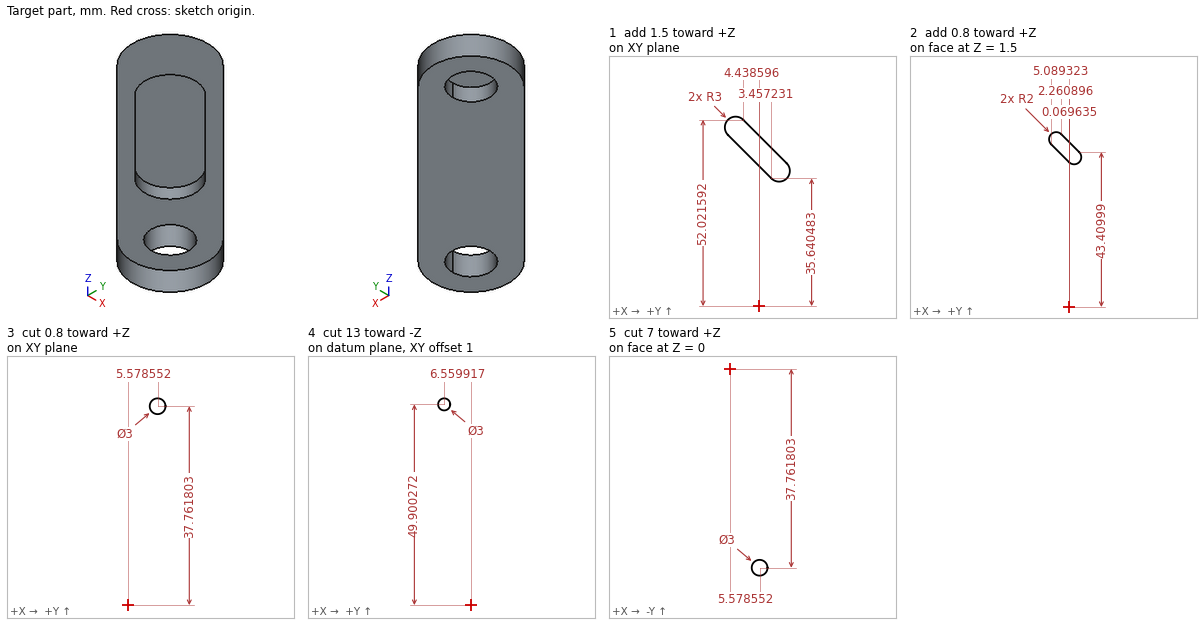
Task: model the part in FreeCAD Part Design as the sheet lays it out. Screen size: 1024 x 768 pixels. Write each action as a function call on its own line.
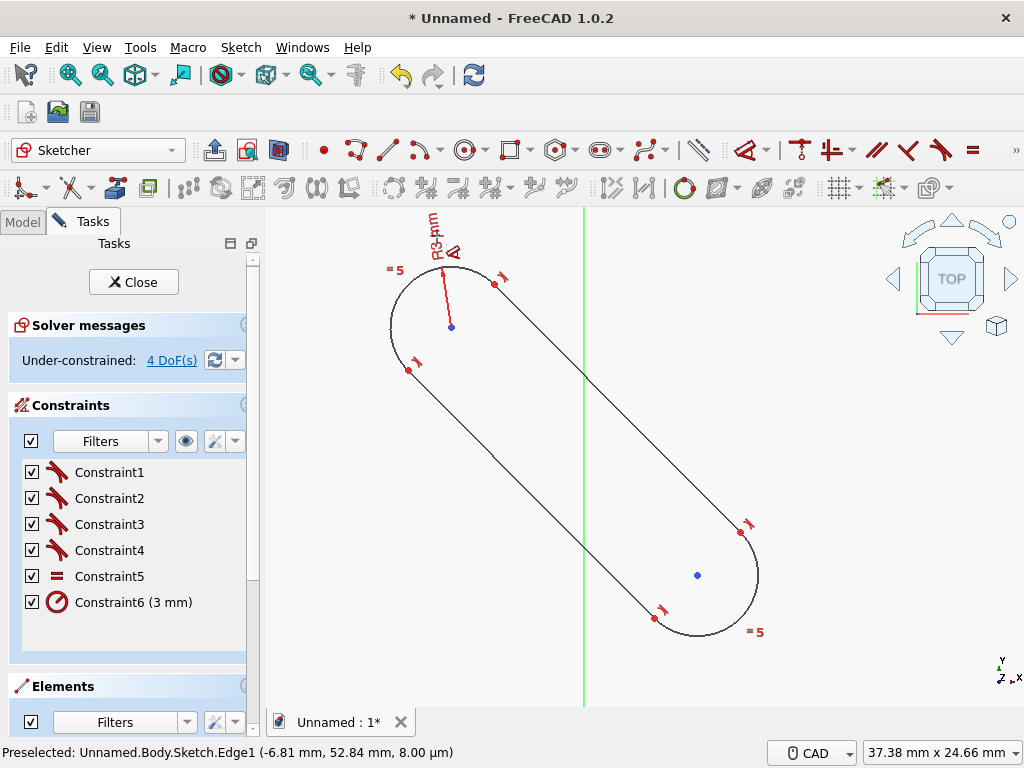
click(494, 285)
click(539, 251)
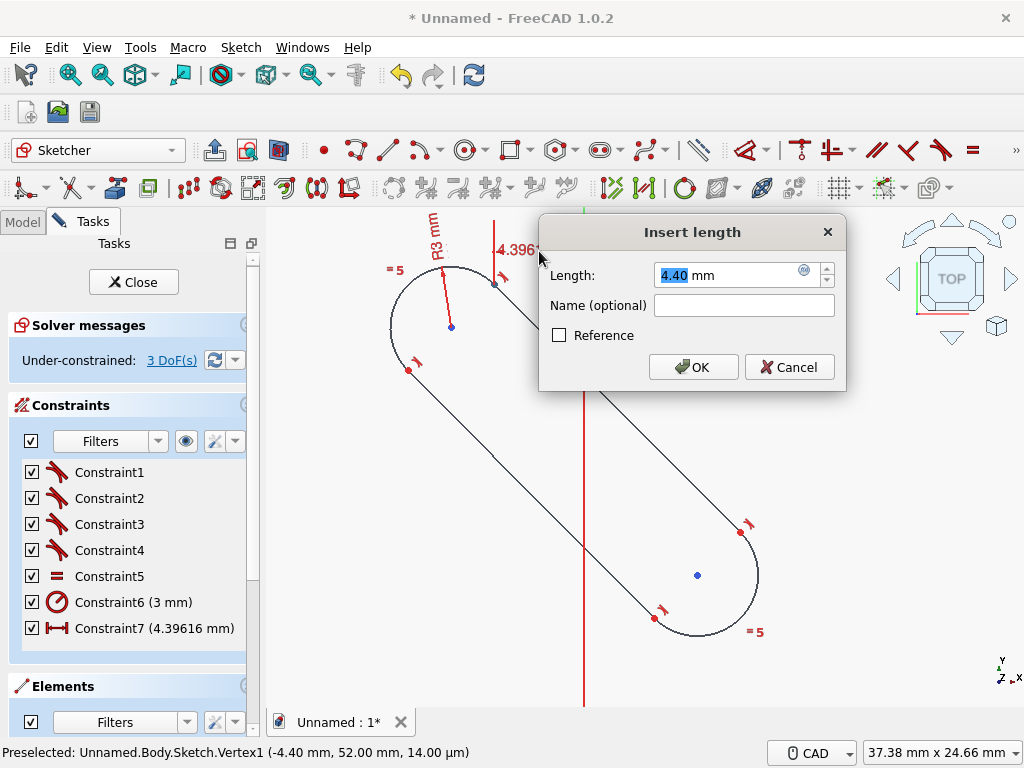
text(4.438596)
key(Return)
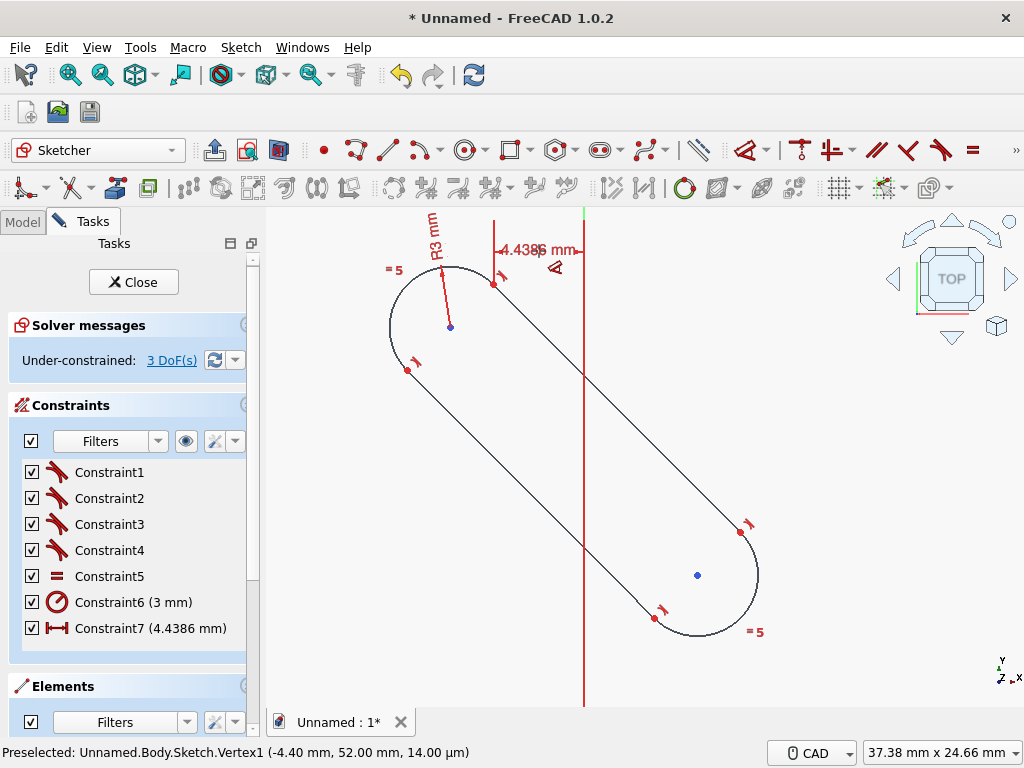
click(654, 618)
click(644, 584)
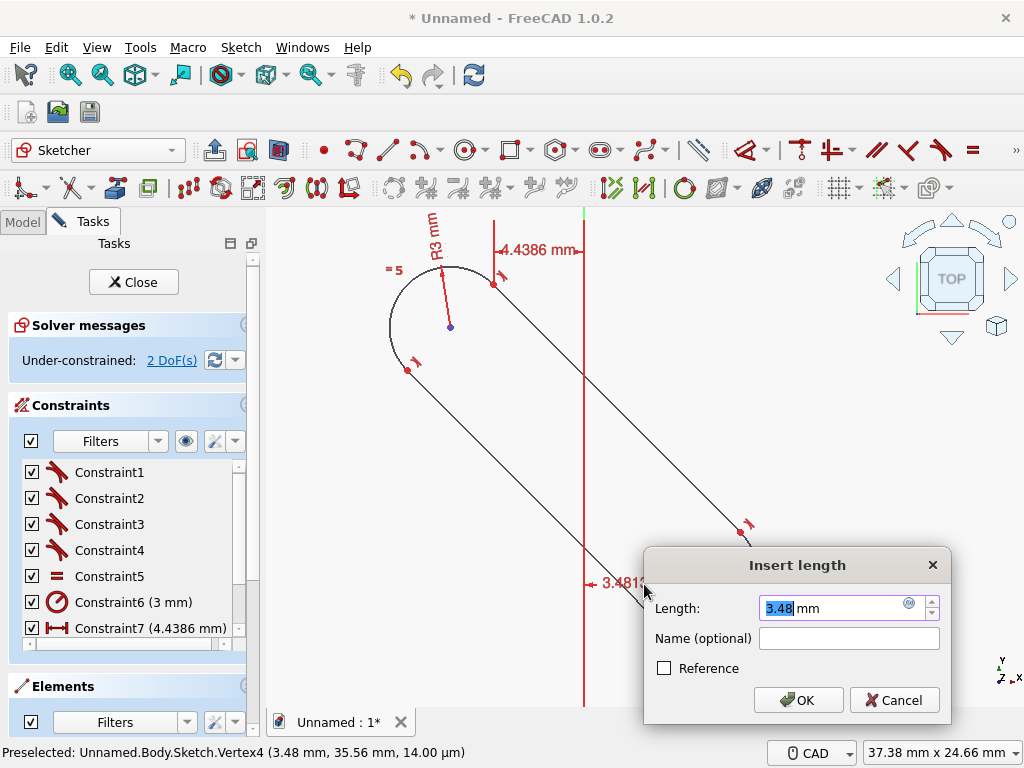
text(3.457231)
key(Return)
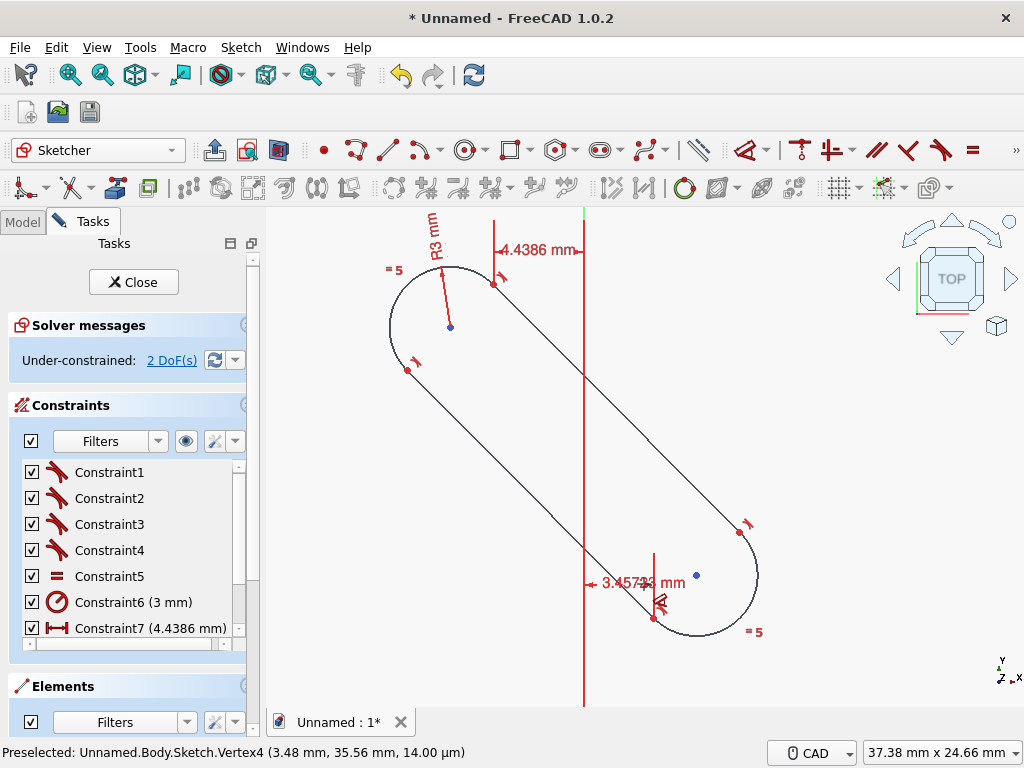
click(494, 285)
click(460, 482)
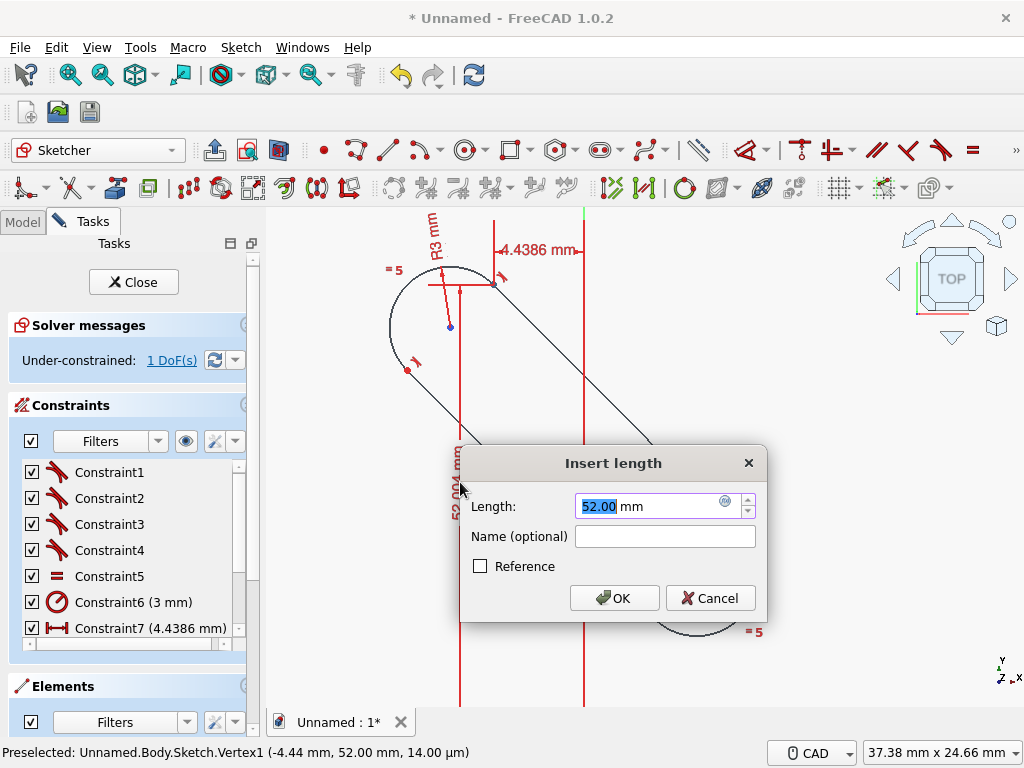
text(52.021592)
key(Return)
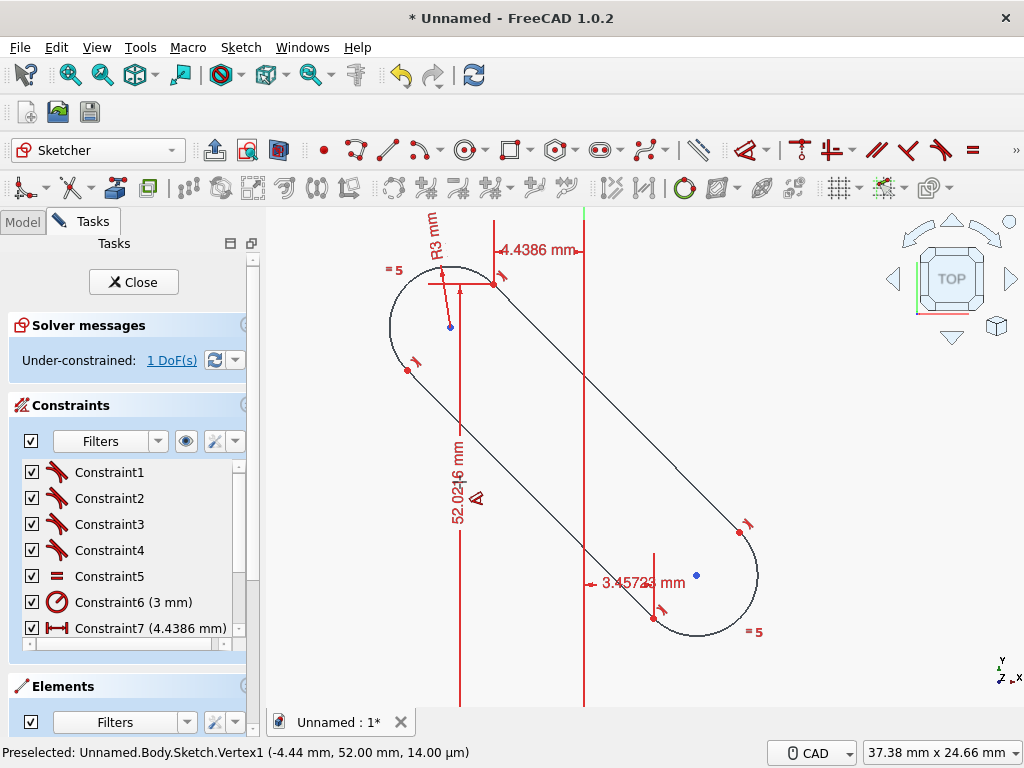
click(654, 618)
click(688, 649)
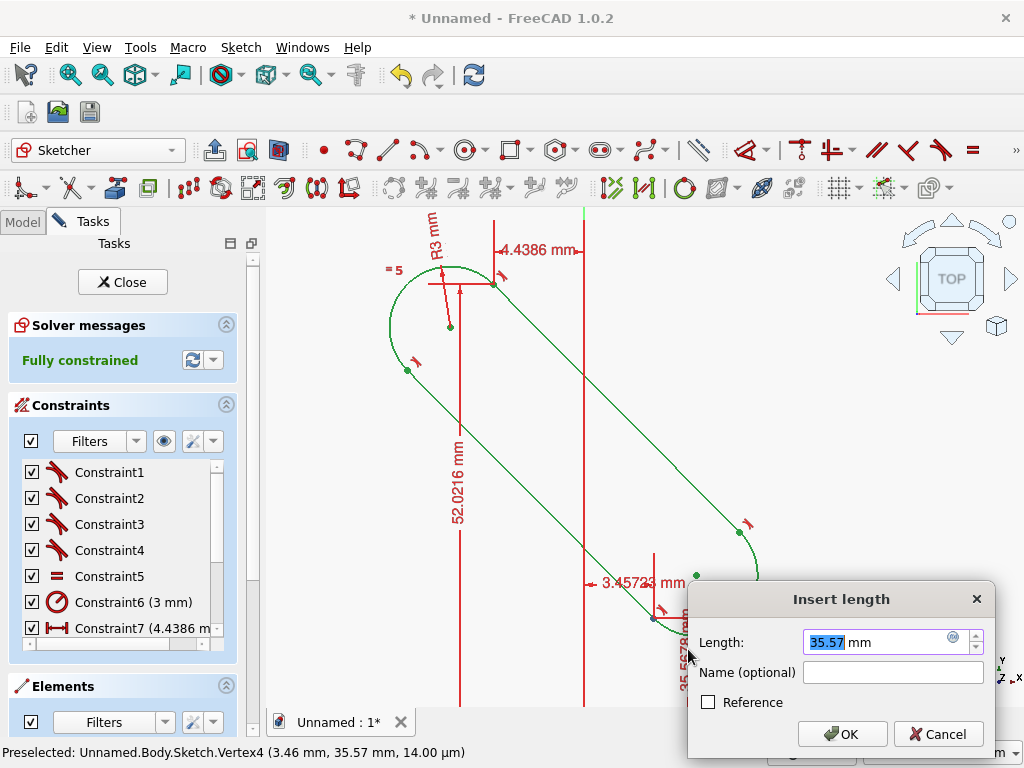
text(35.640483)
key(Return)
key(Escape)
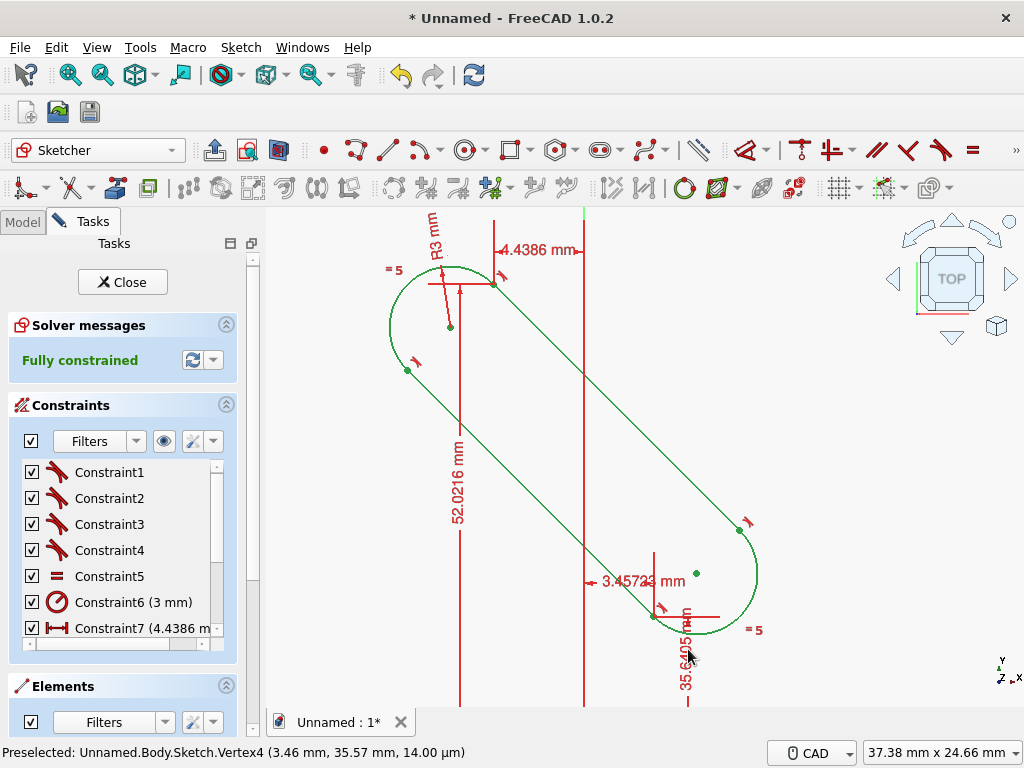
click(123, 282)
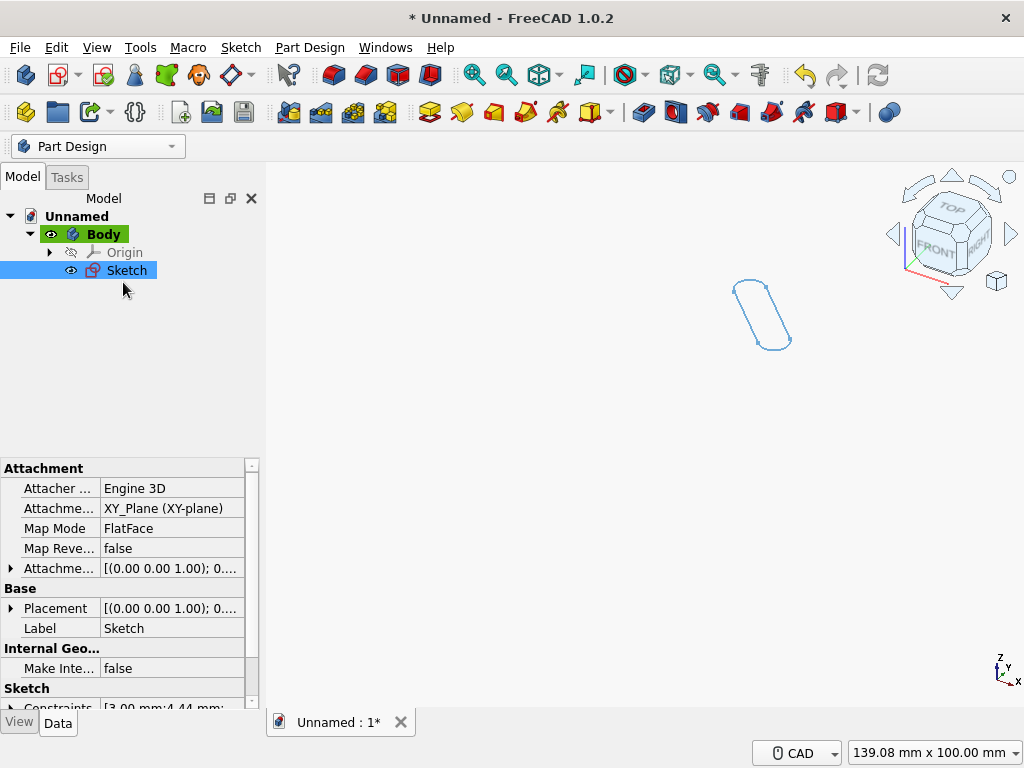
click(430, 112)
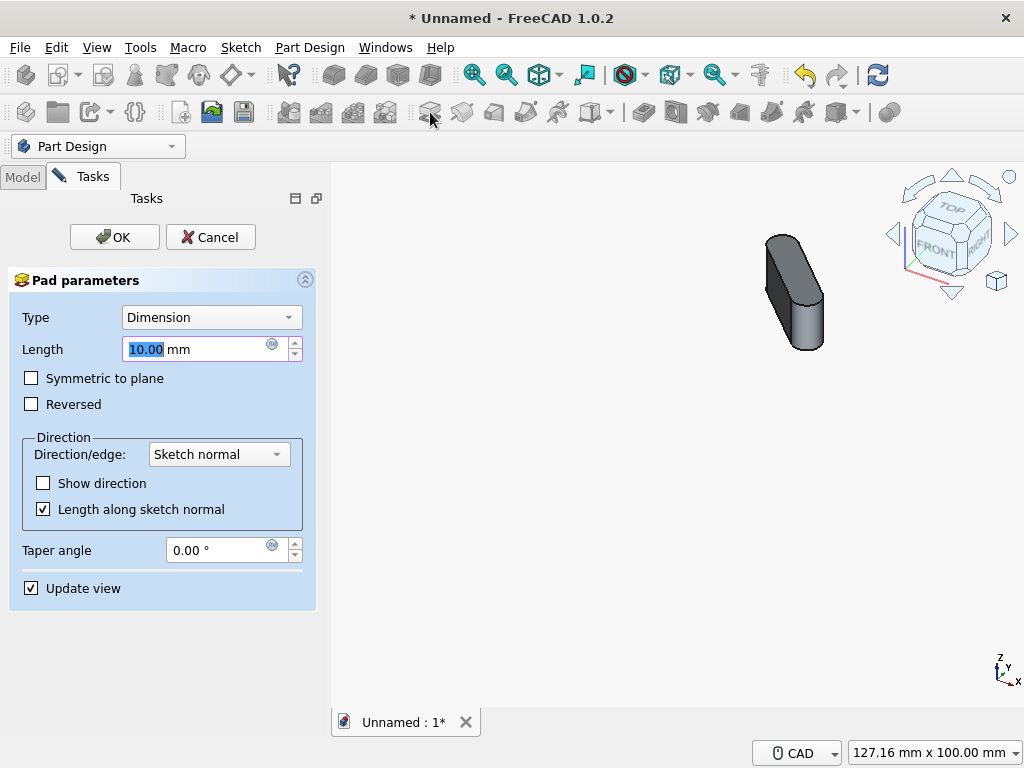
text(1.5)
key(Tab)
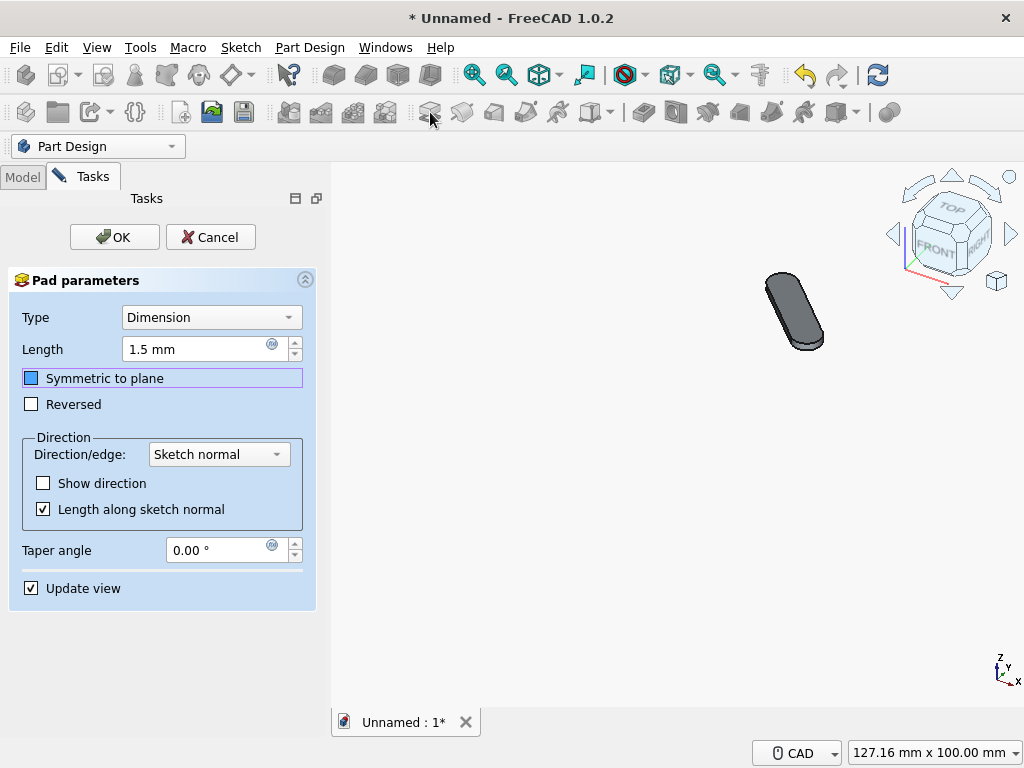
click(115, 237)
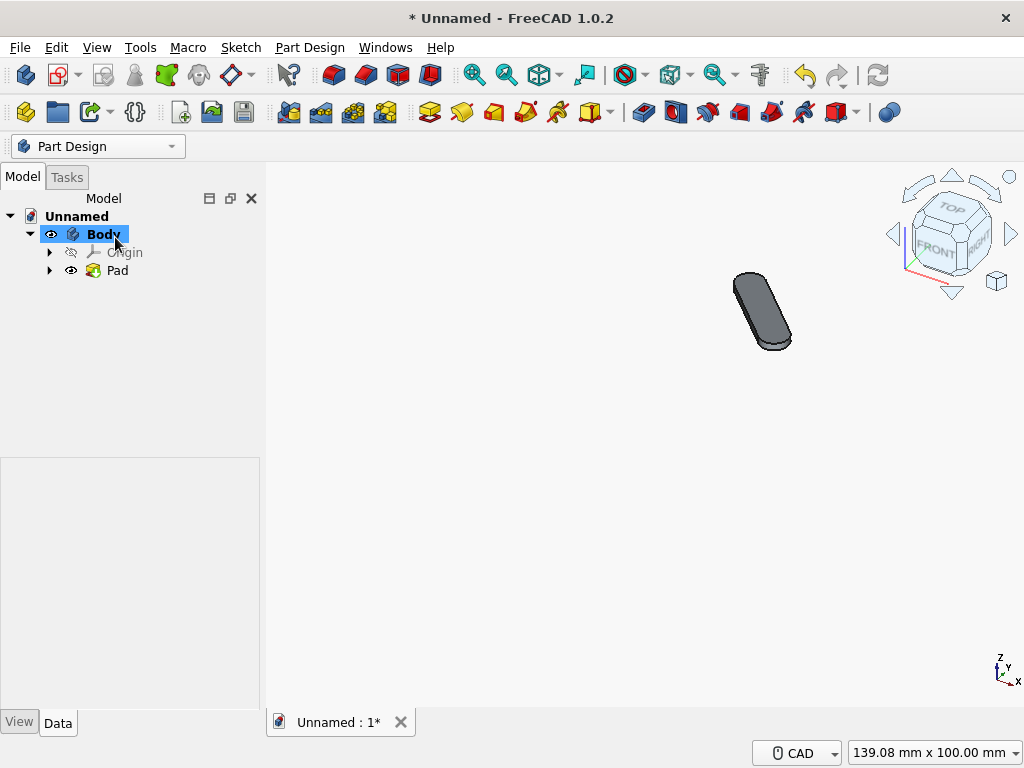
click(476, 76)